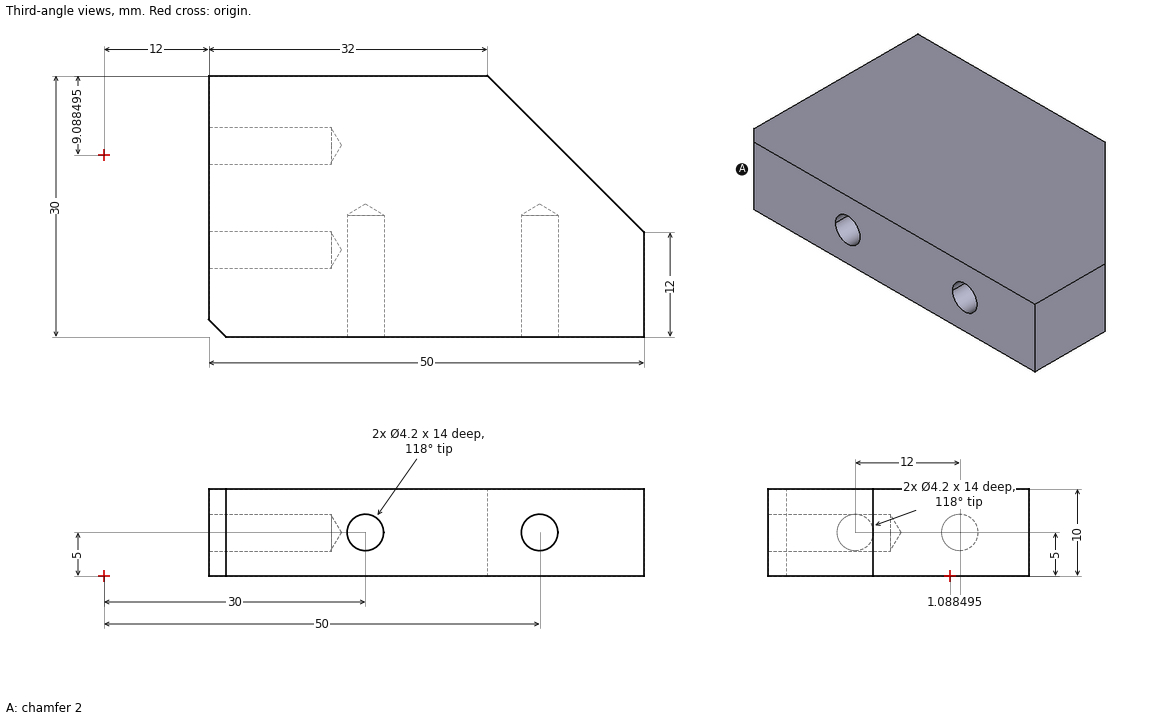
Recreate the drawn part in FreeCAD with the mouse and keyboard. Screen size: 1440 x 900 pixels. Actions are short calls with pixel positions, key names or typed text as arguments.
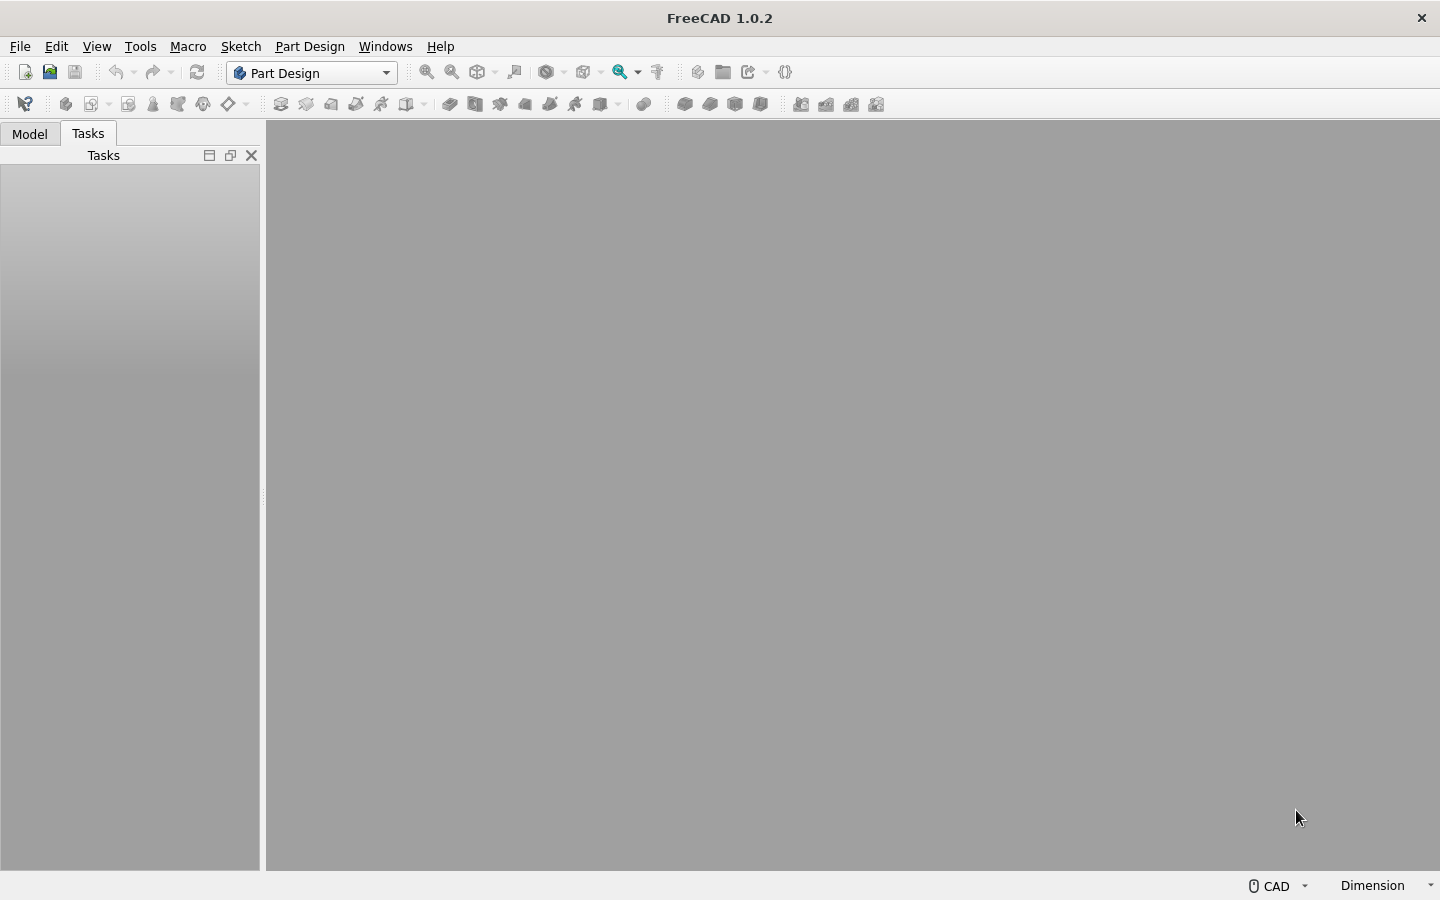
click(25, 72)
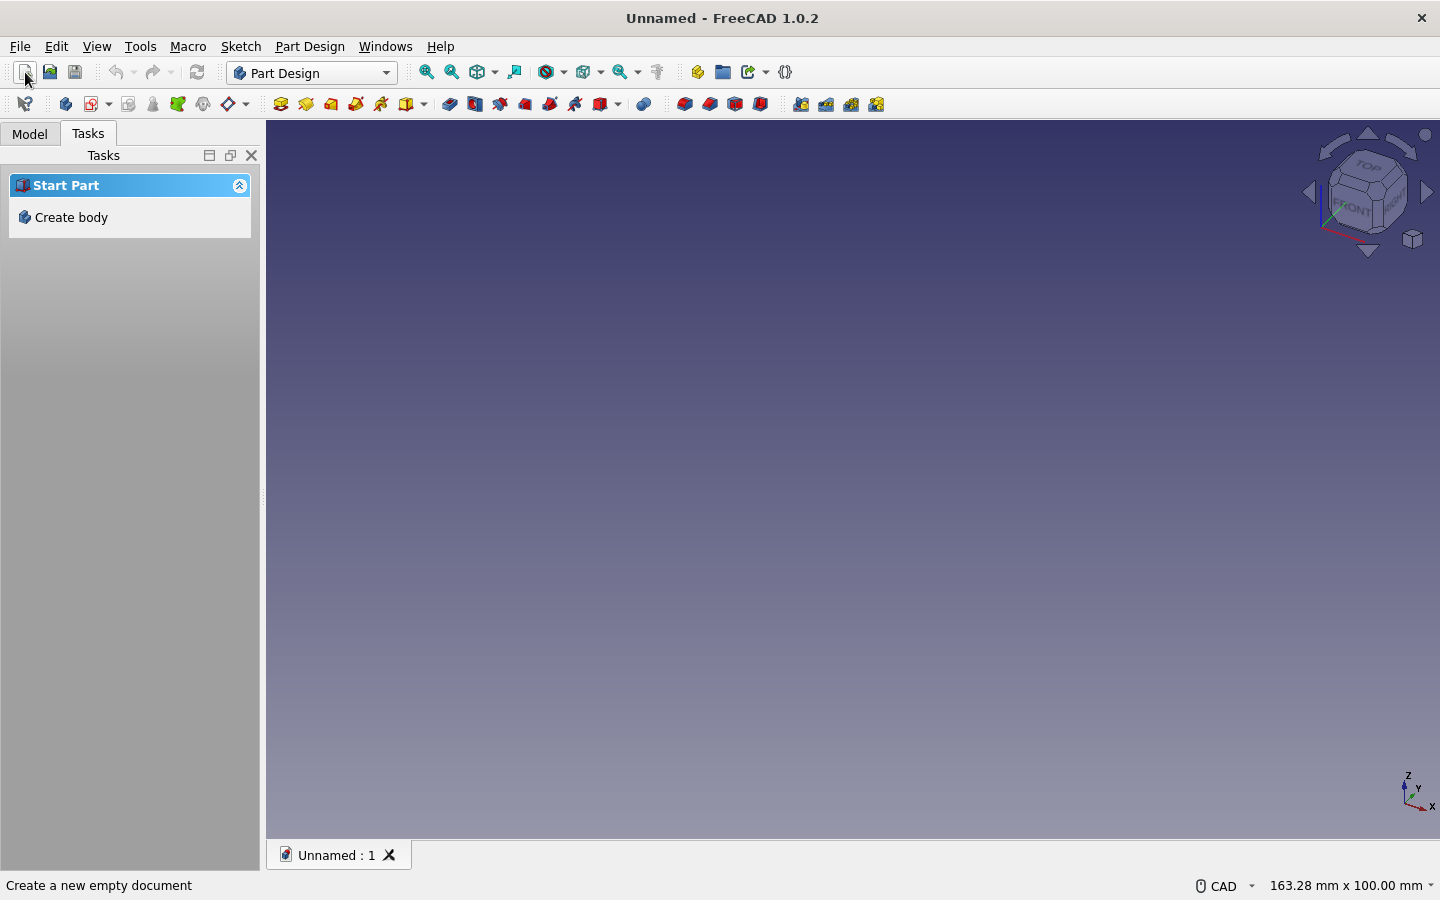
click(90, 104)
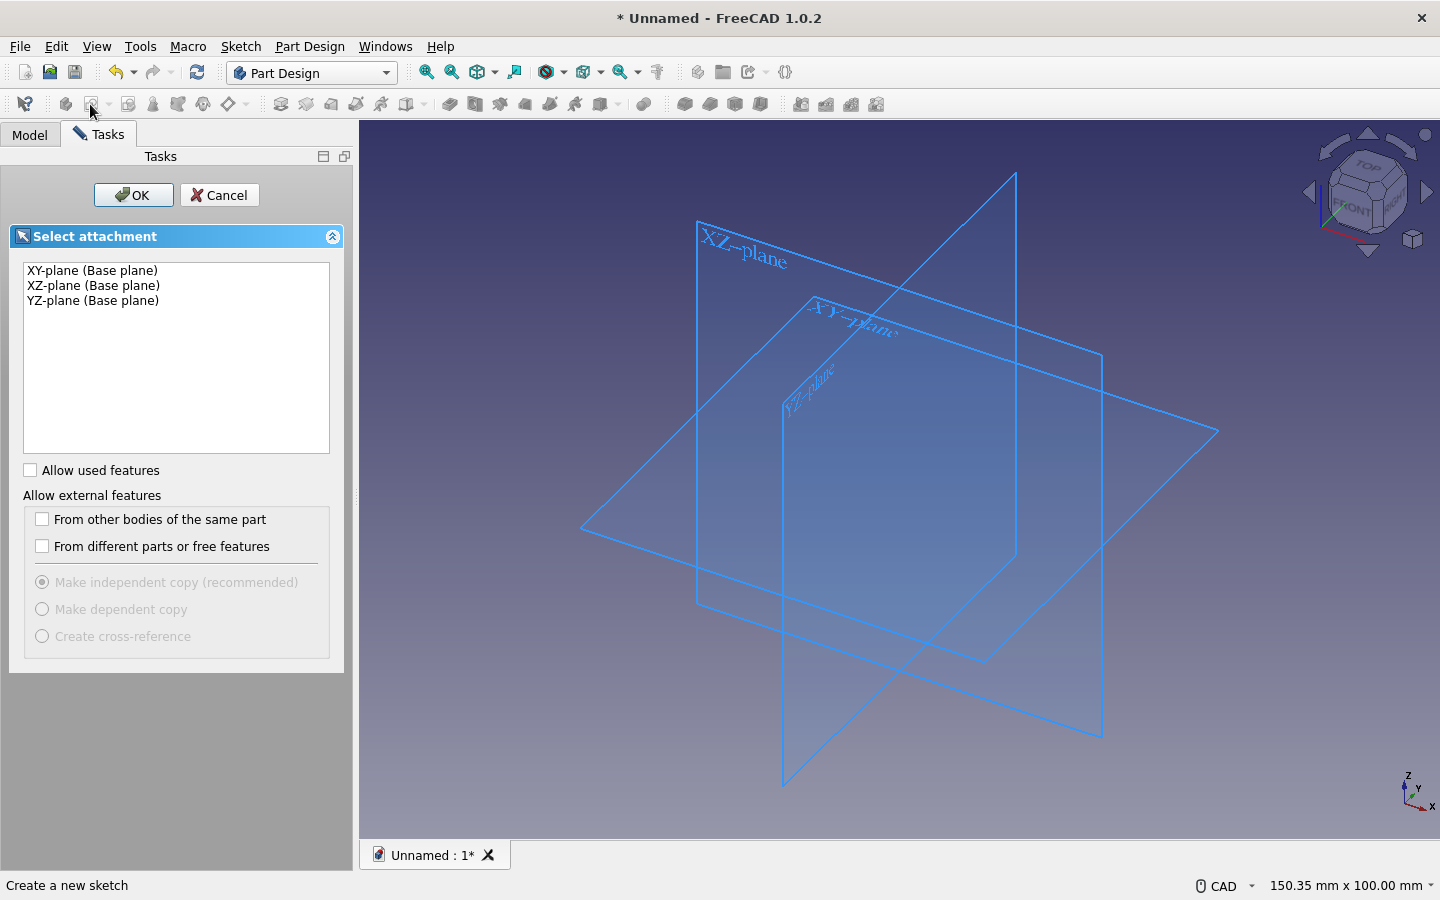
click(84, 270)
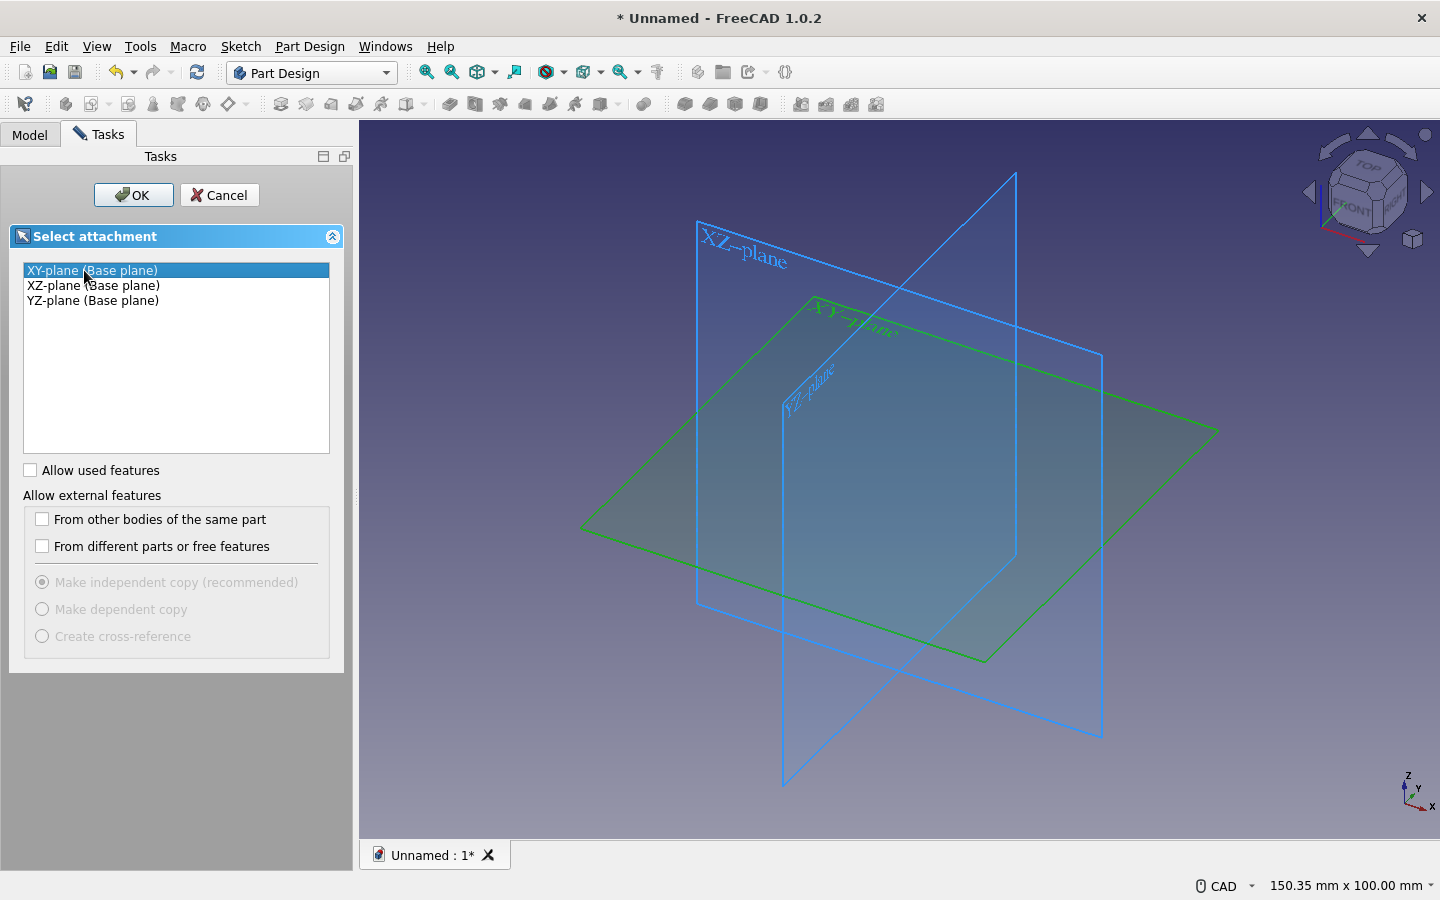
click(134, 195)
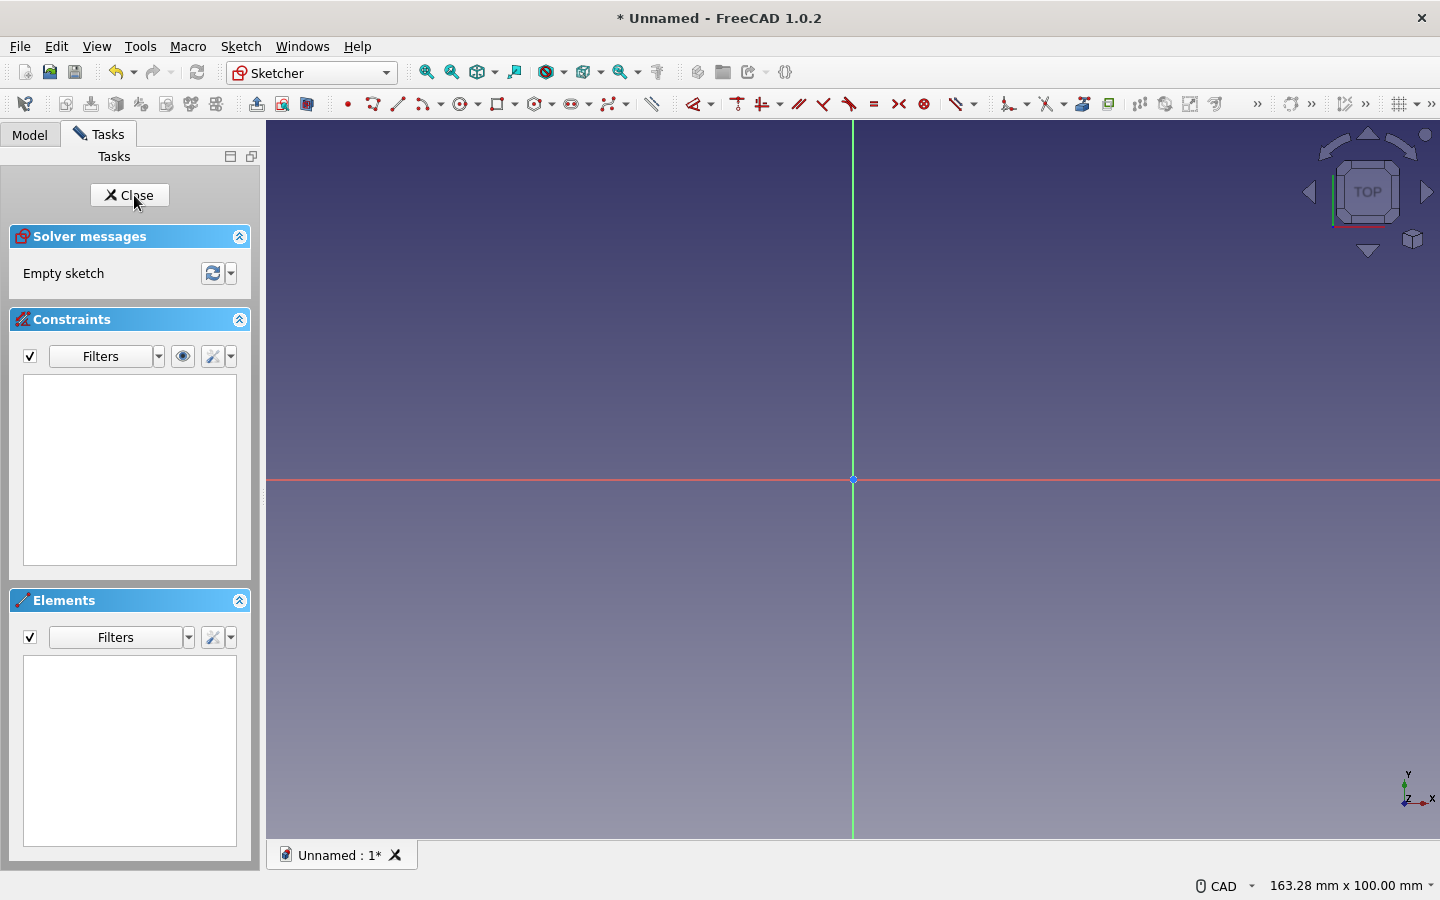
scroll(294, 288, down, 1)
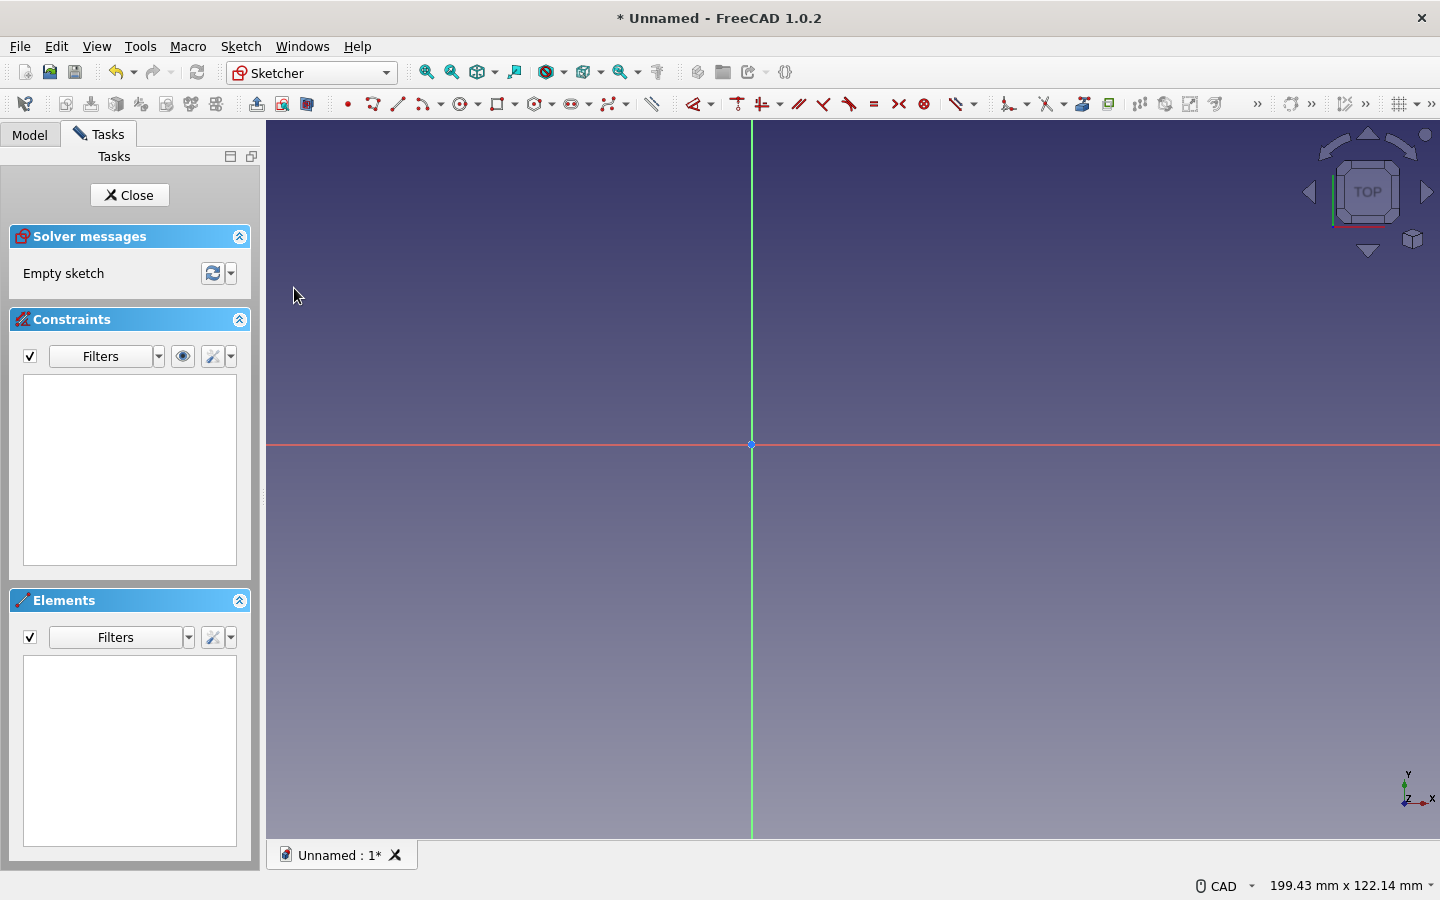
scroll(1116, 480, up, 3)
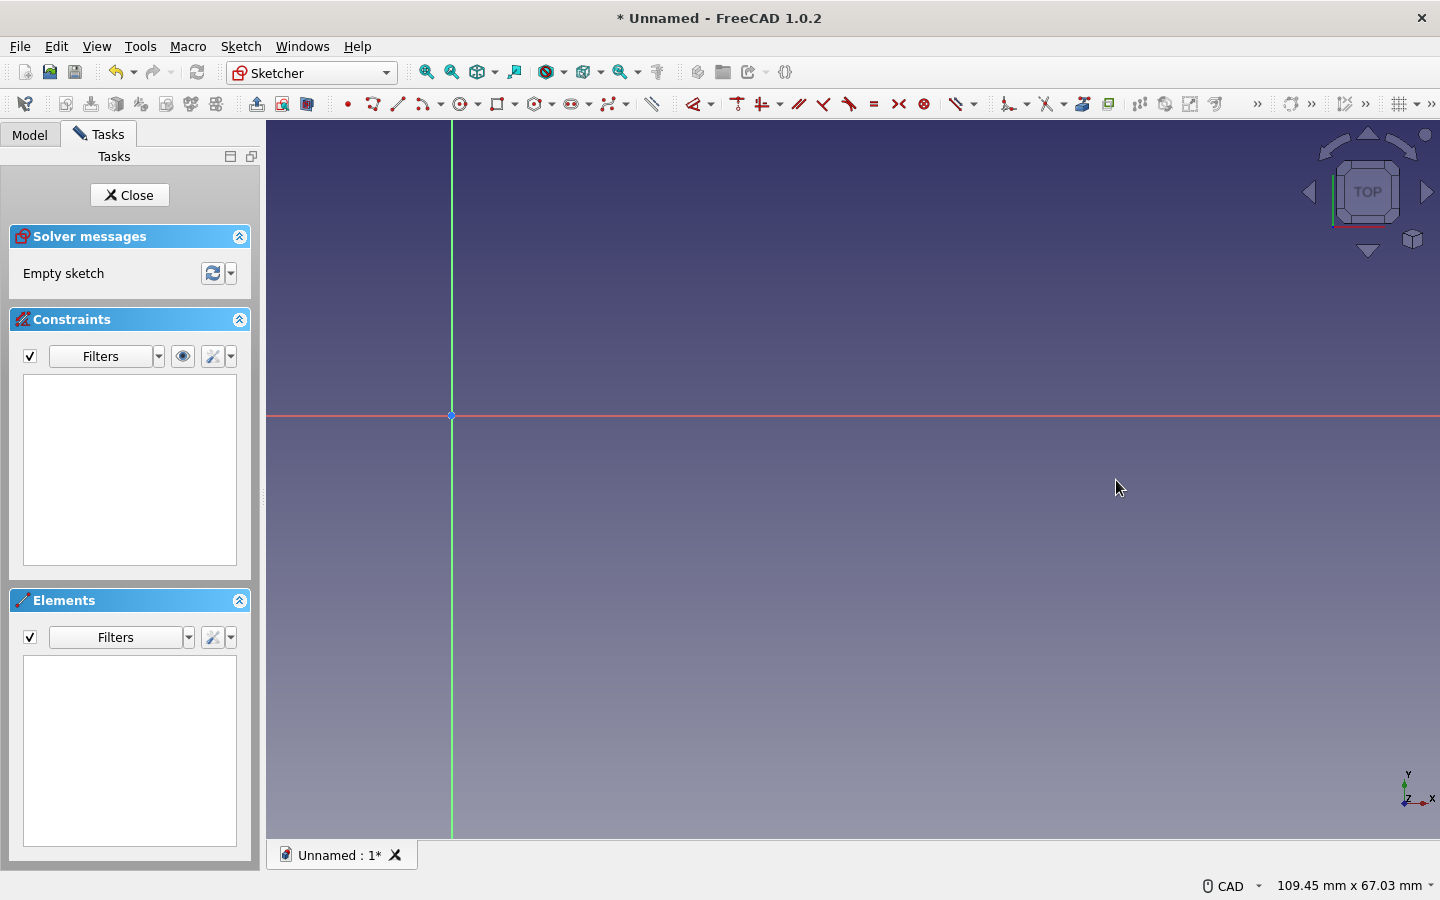
click(373, 104)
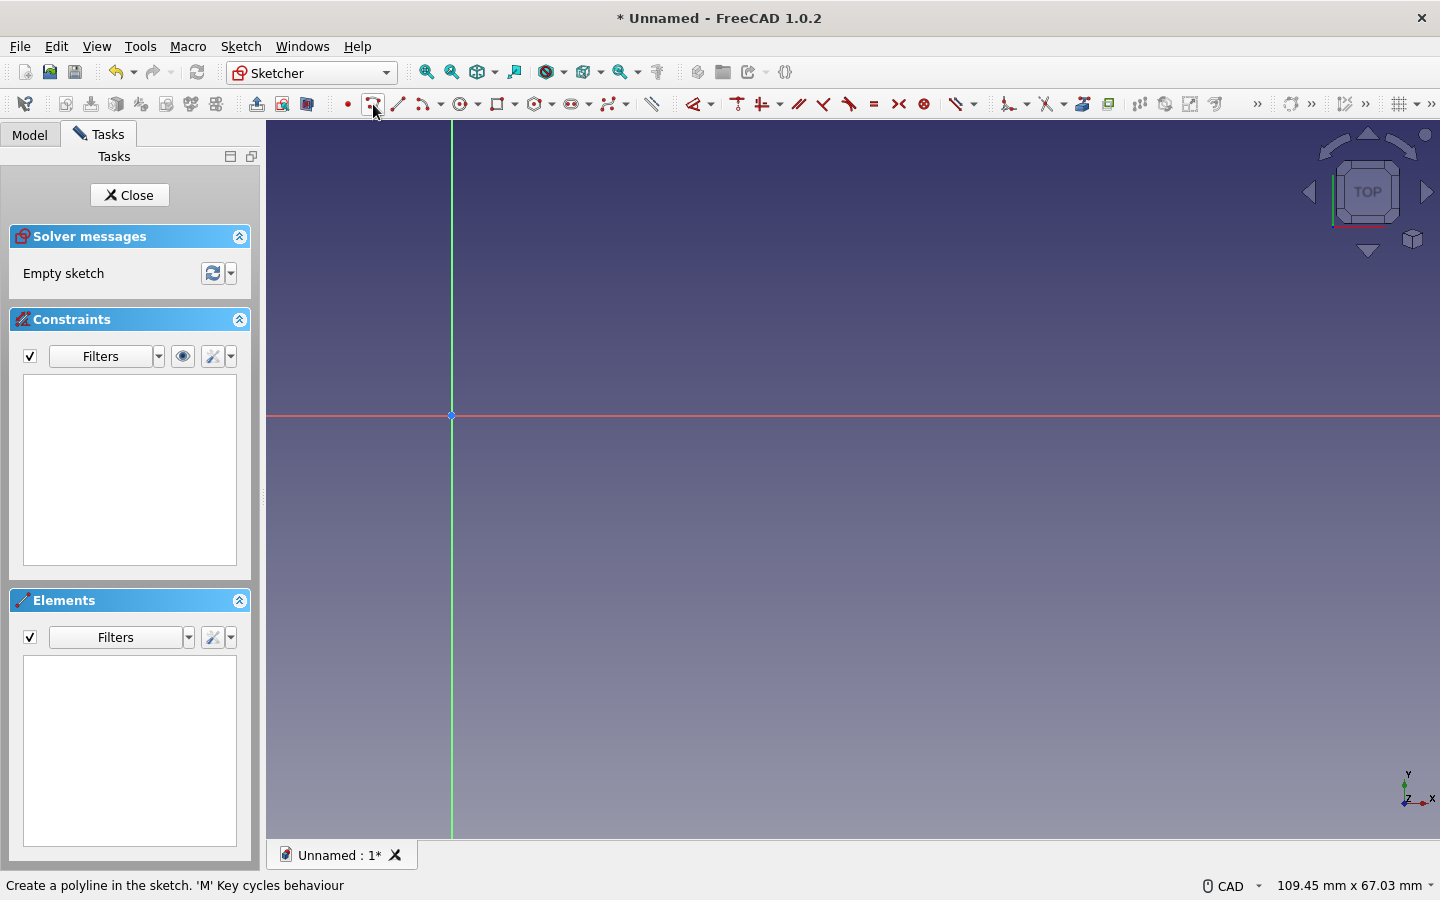
click(580, 318)
click(580, 640)
click(1117, 640)
click(1117, 511)
click(924, 318)
click(580, 319)
key(Escape)
key(Escape)